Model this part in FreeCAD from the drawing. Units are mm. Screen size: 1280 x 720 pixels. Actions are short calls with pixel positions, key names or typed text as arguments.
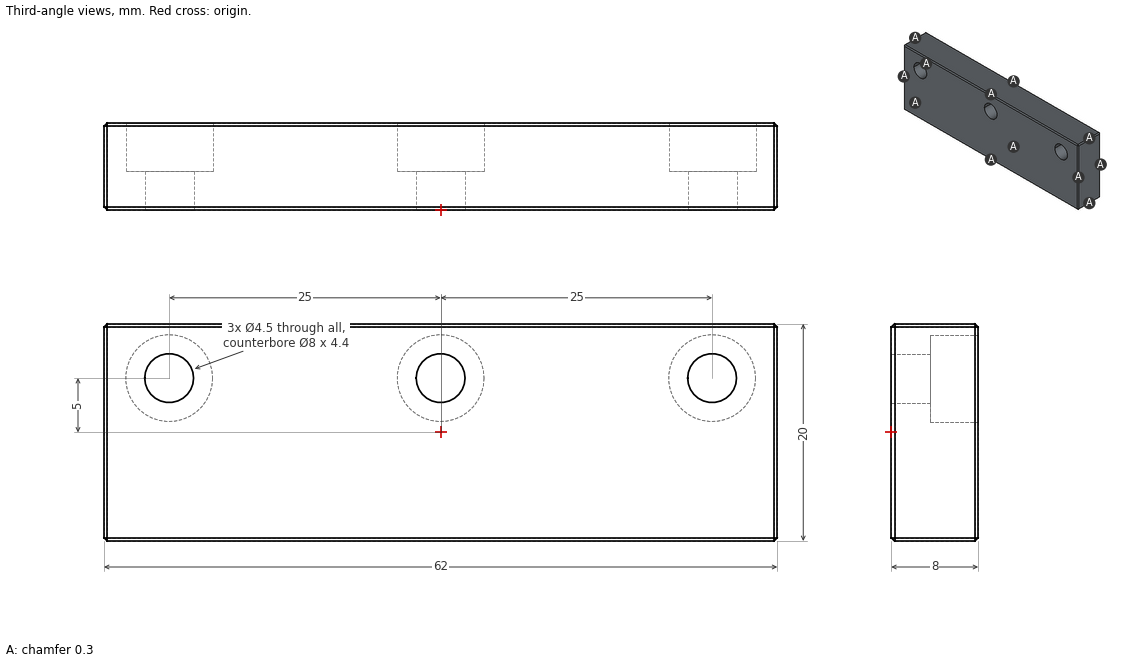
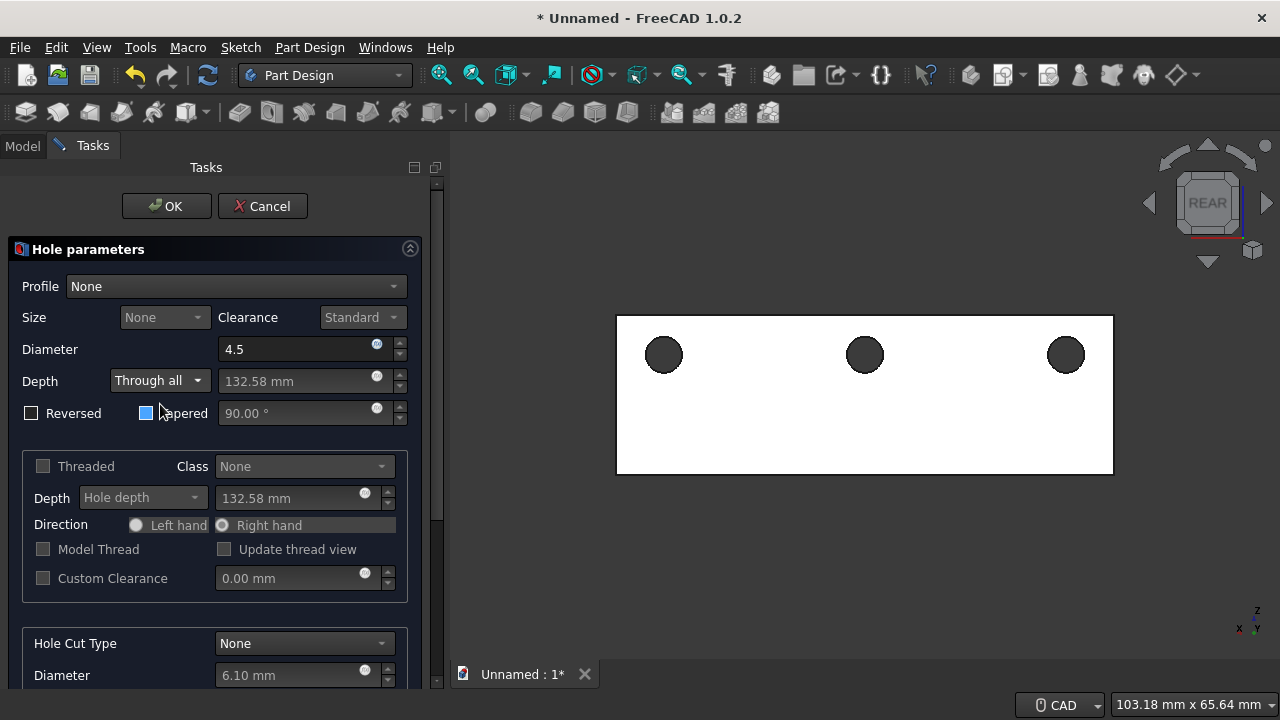
click(306, 644)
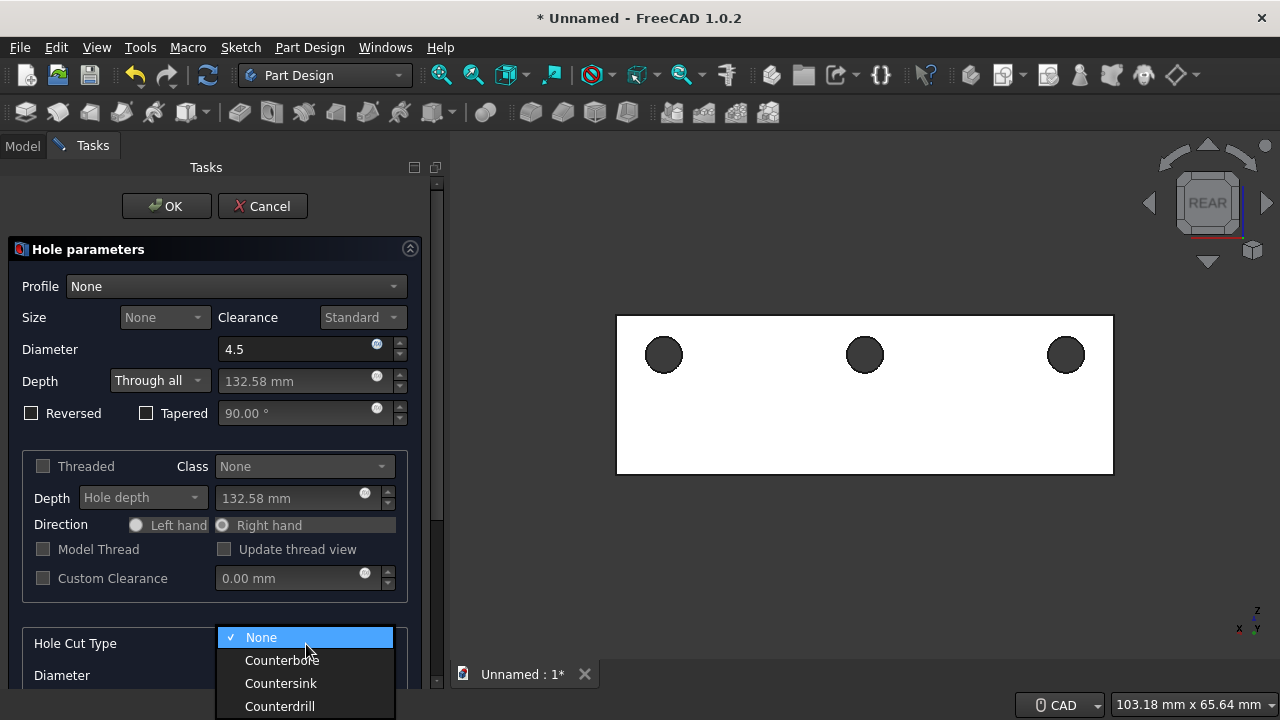
click(304, 660)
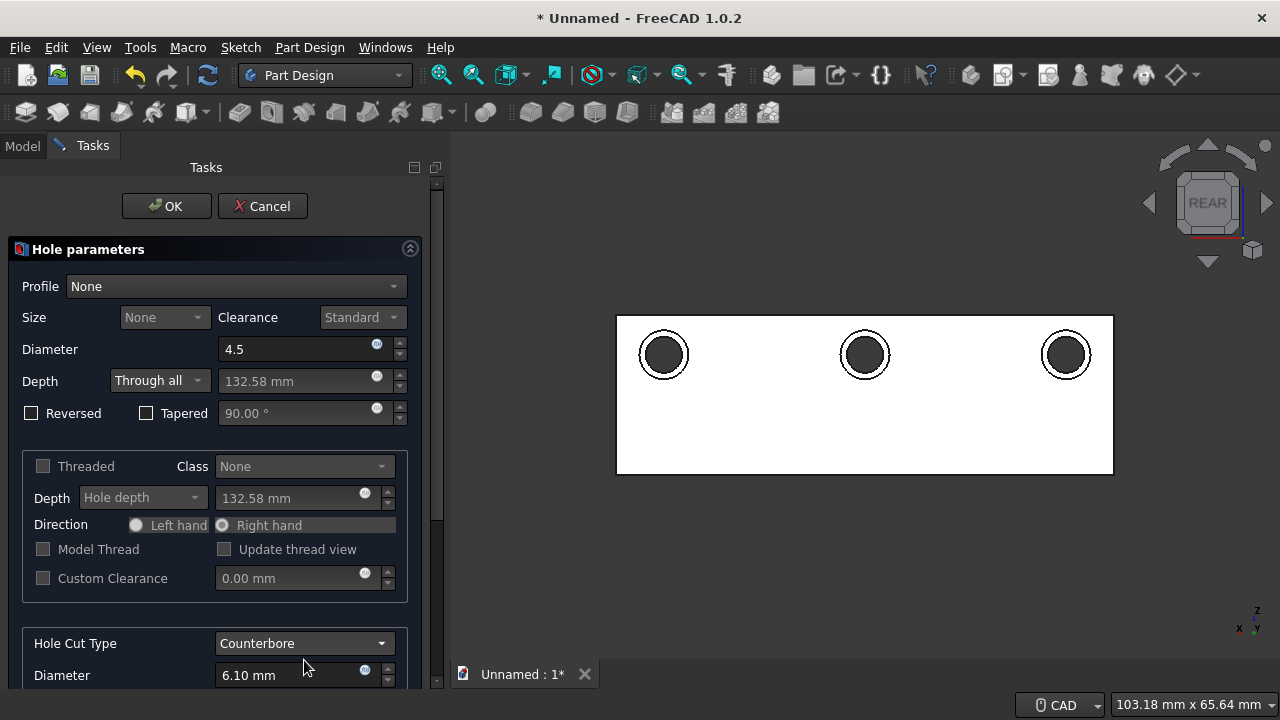
triple_click(298, 675)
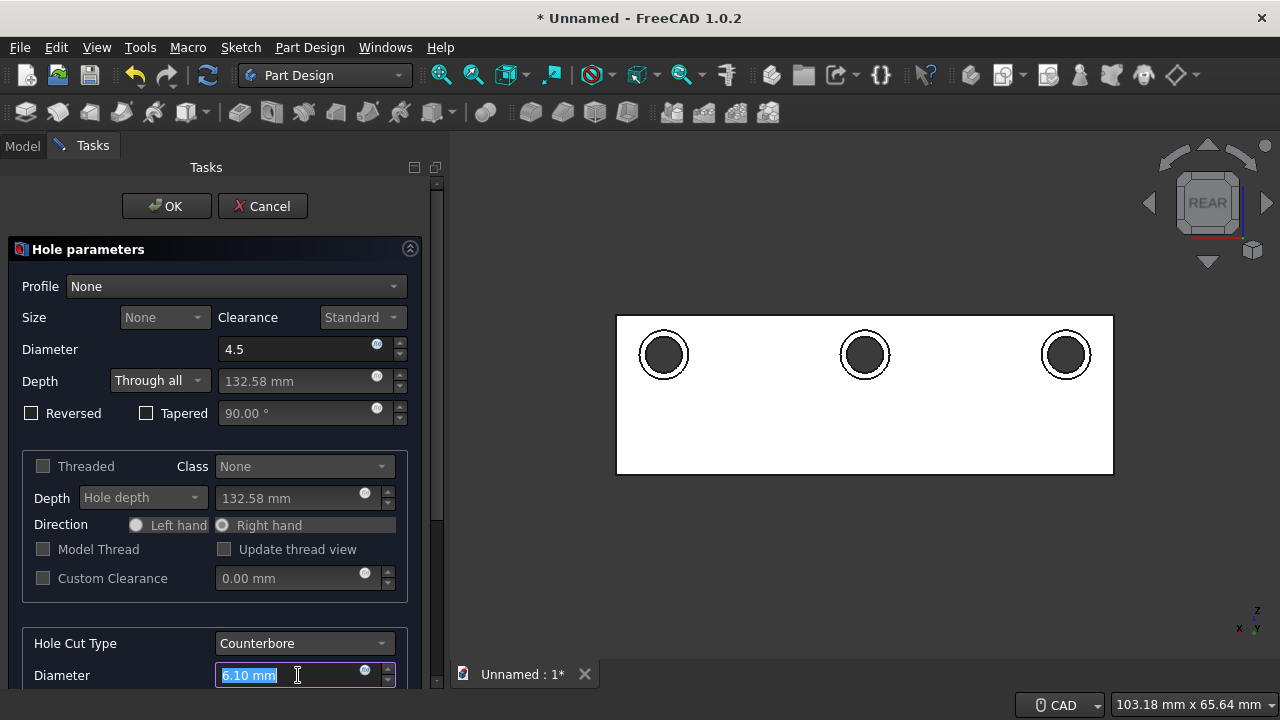
text(8)
key(Tab)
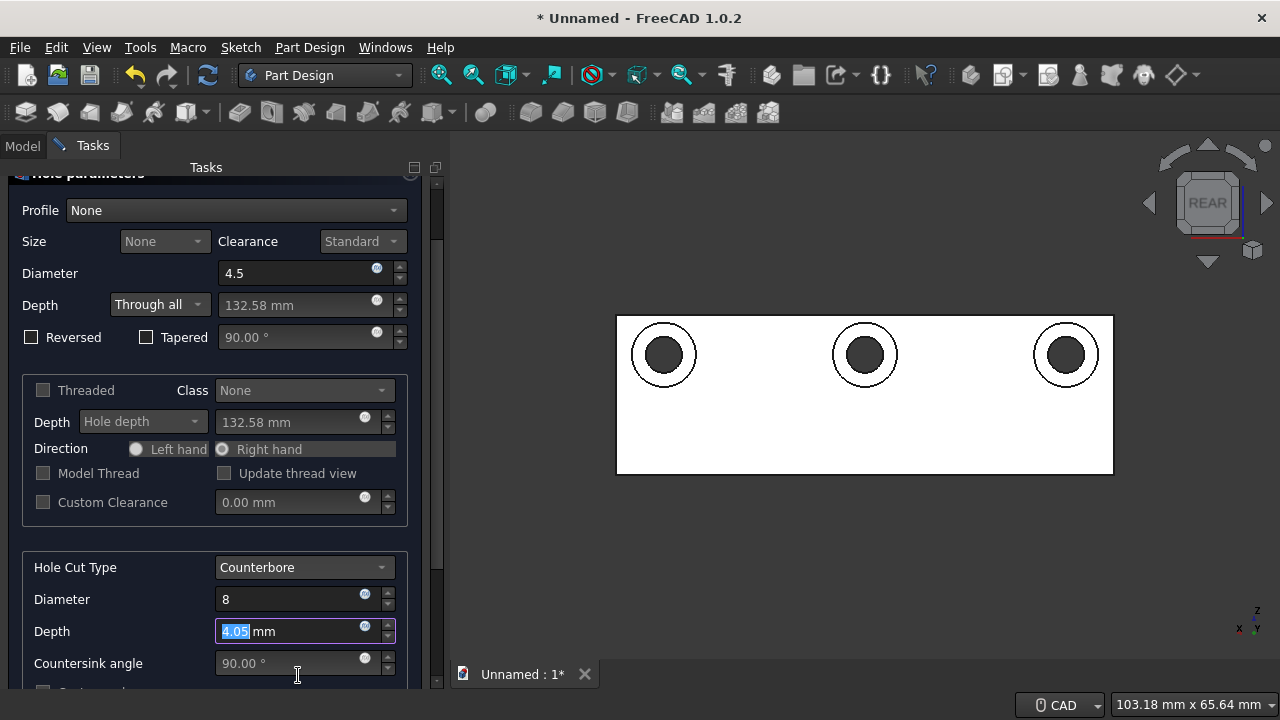
text(4.4)
key(Tab)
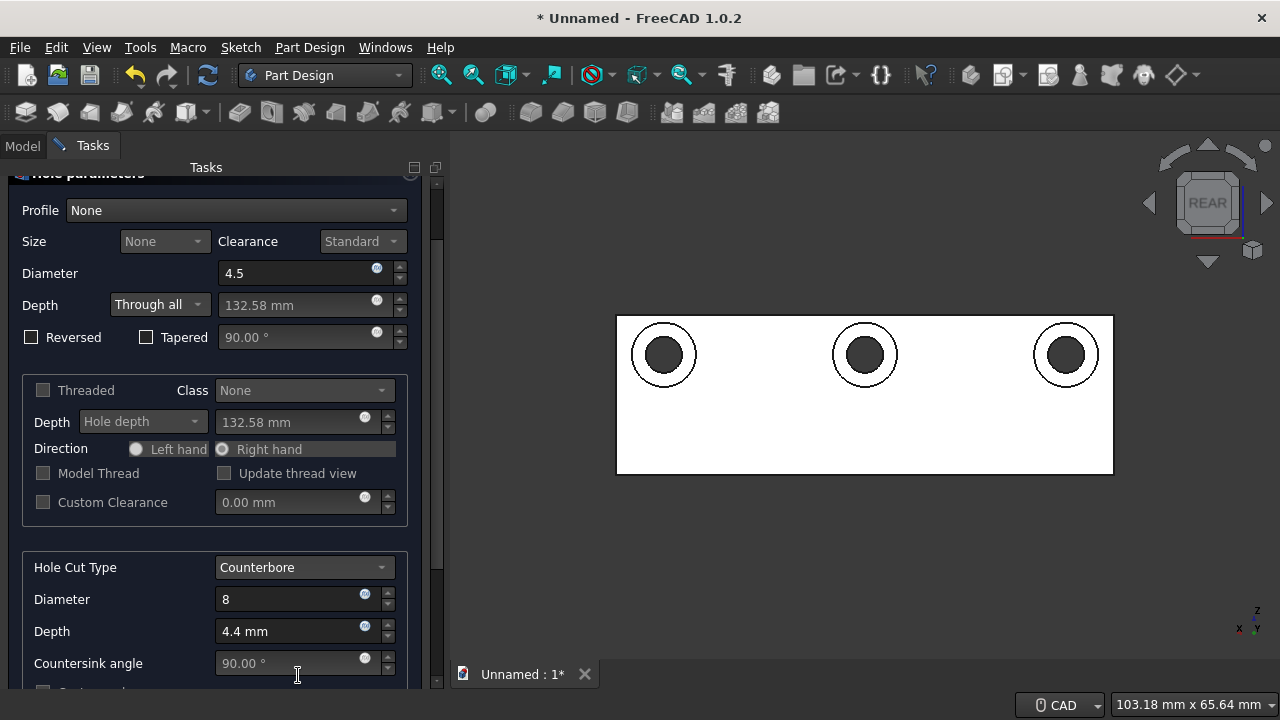
scroll(437, 432, up, 3)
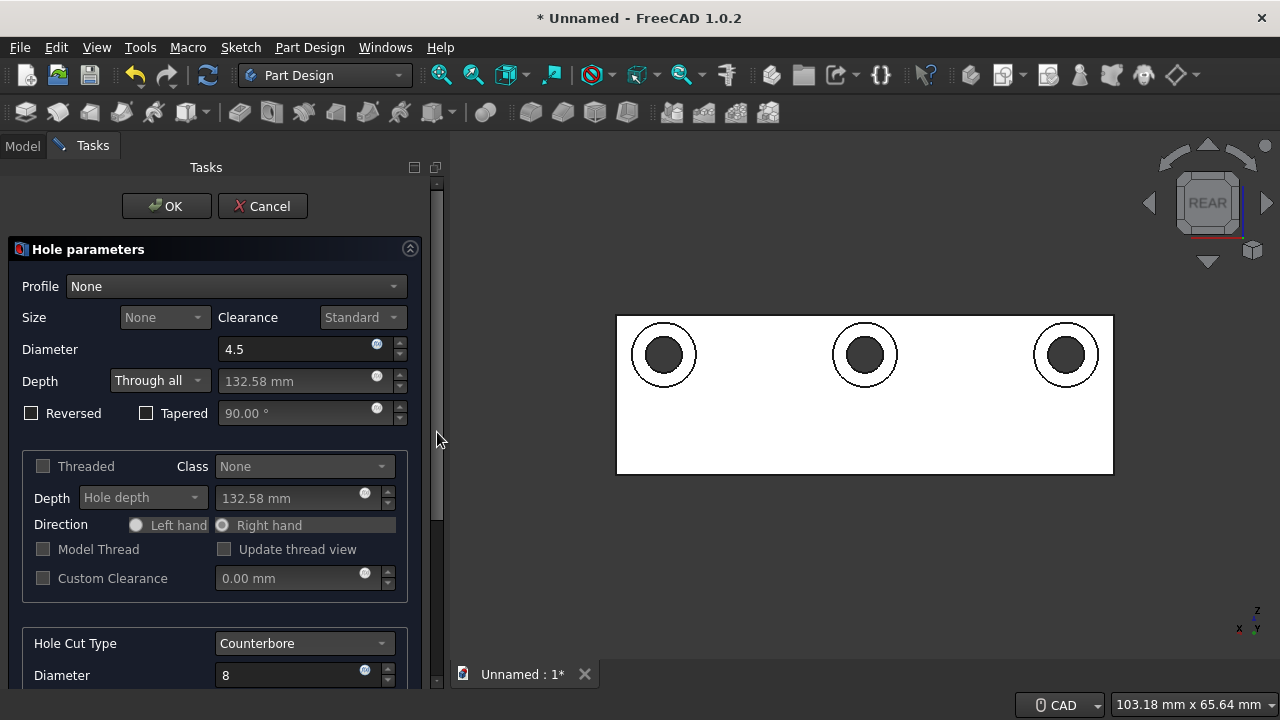
click(167, 206)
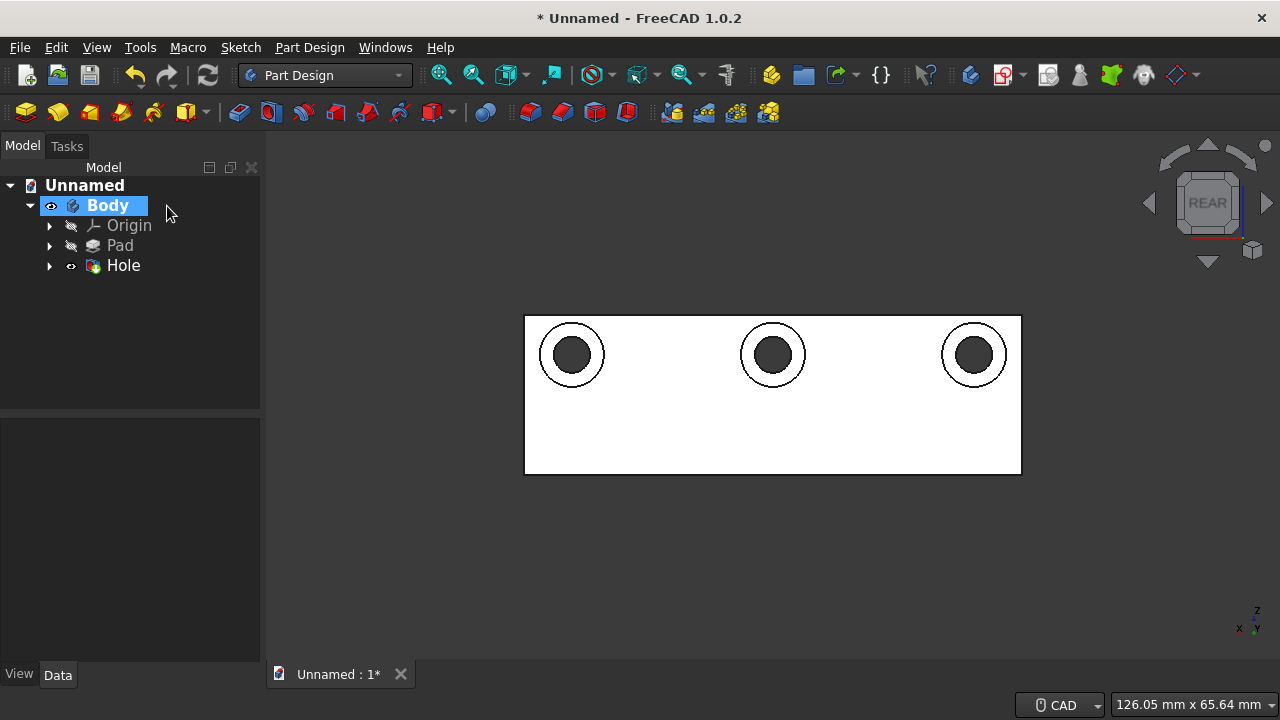
click(1022, 394)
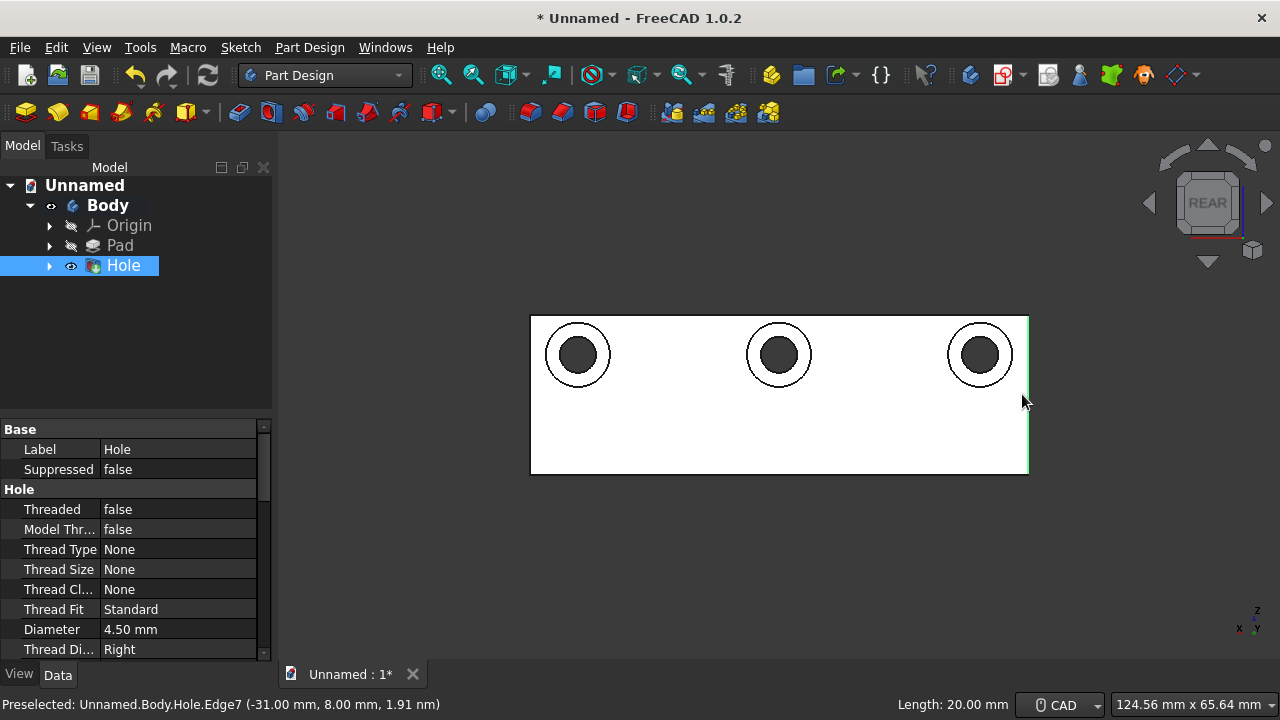
key(0)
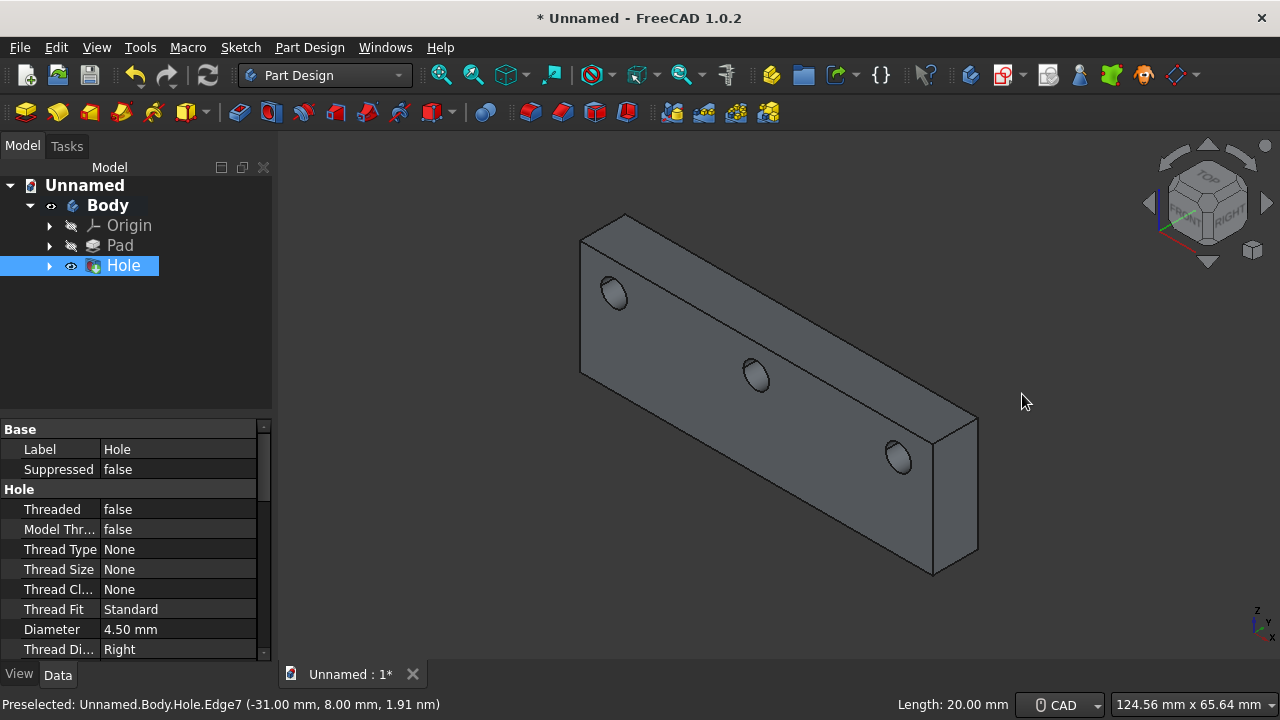
click(930, 416, ctrl)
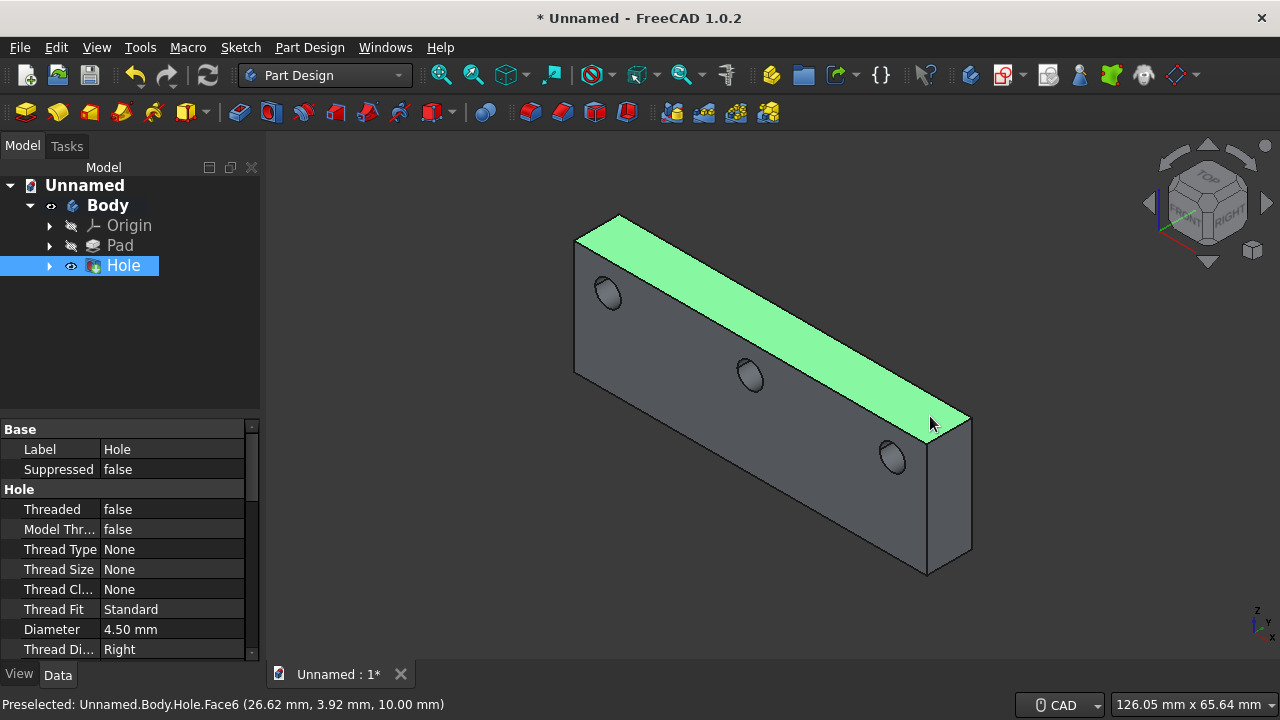
click(927, 509, ctrl)